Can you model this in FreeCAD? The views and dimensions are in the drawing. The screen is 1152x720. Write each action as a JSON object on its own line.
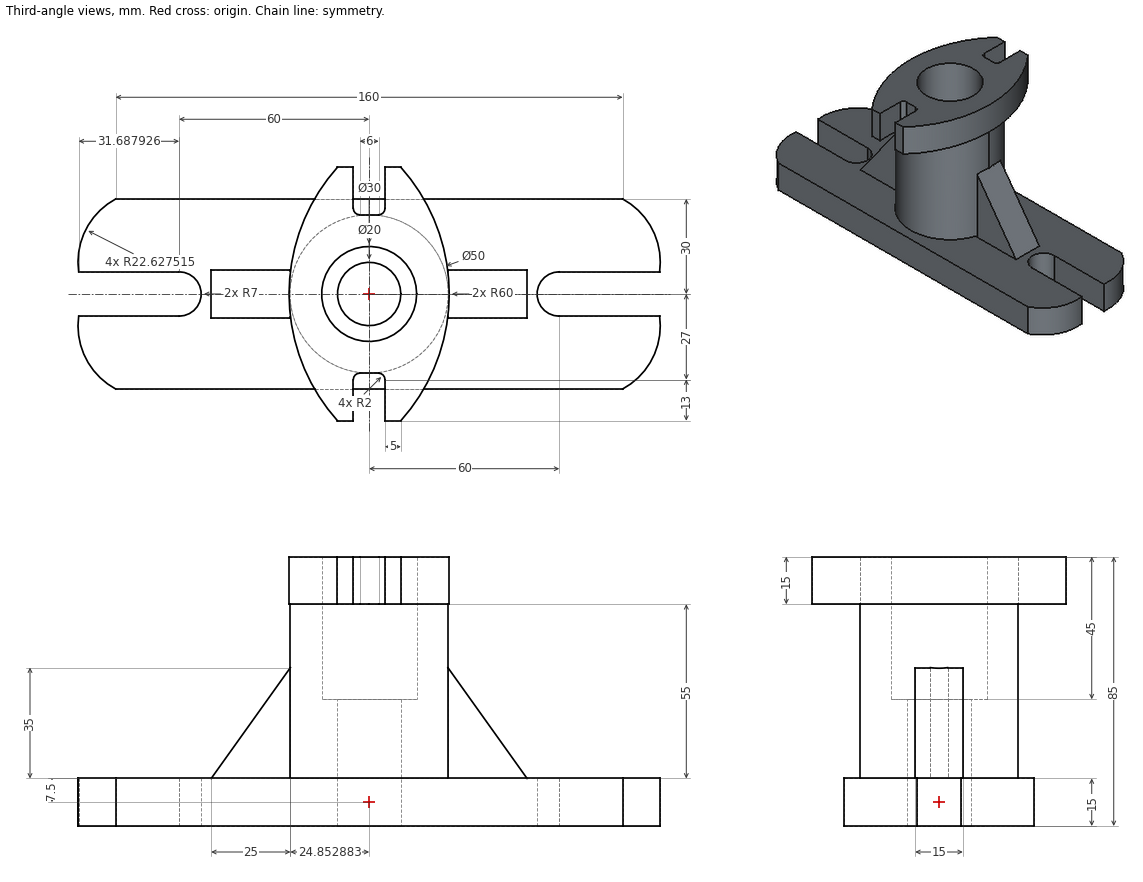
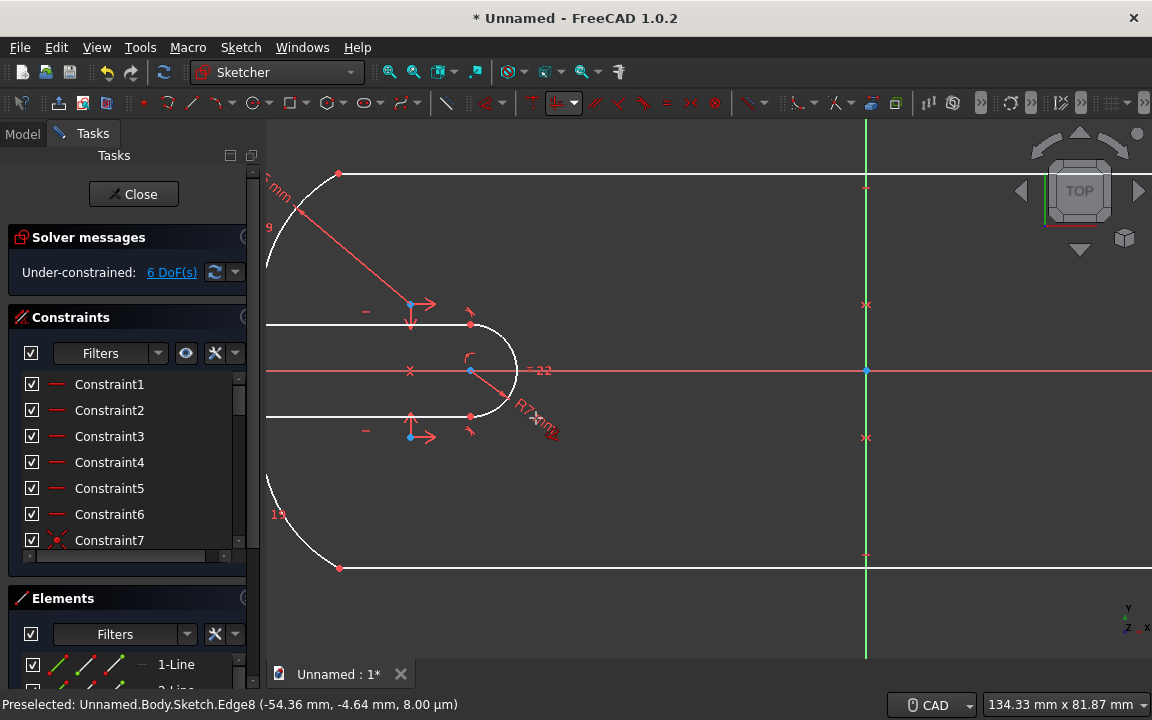
{"action": "left_click", "coordinate": [655, 174]}
{"action": "left_click", "coordinate": [663, 208]}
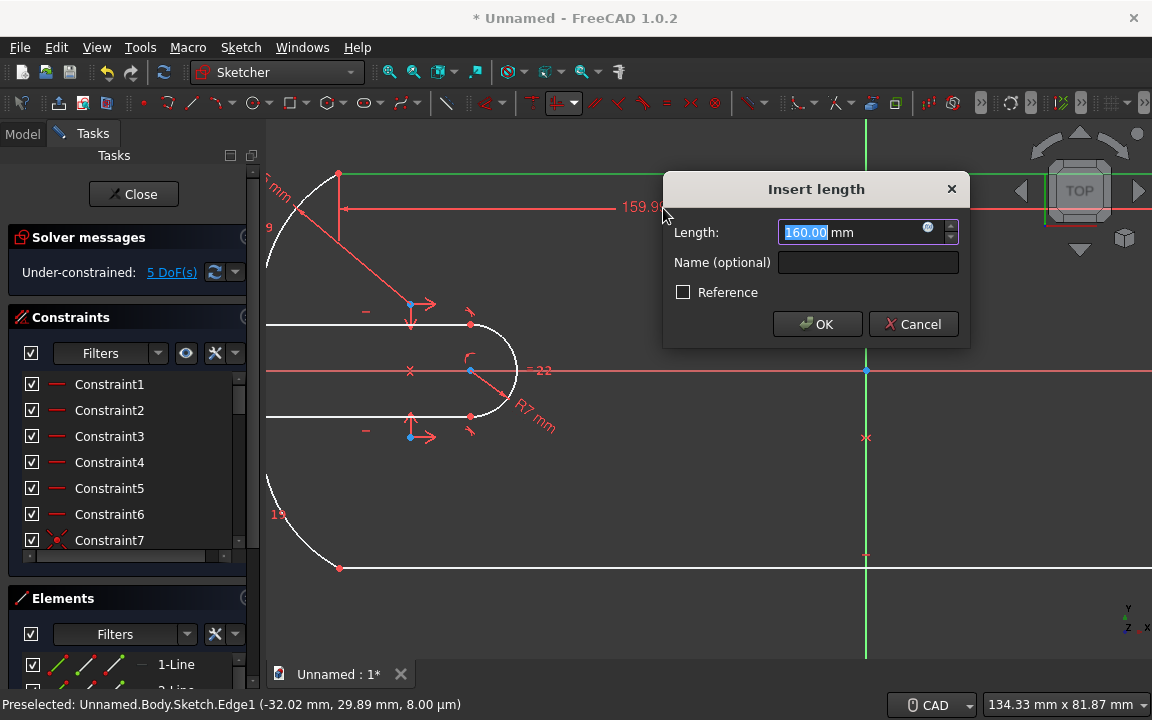
{"action": "type", "text": "160"}
{"action": "key", "text": "Return"}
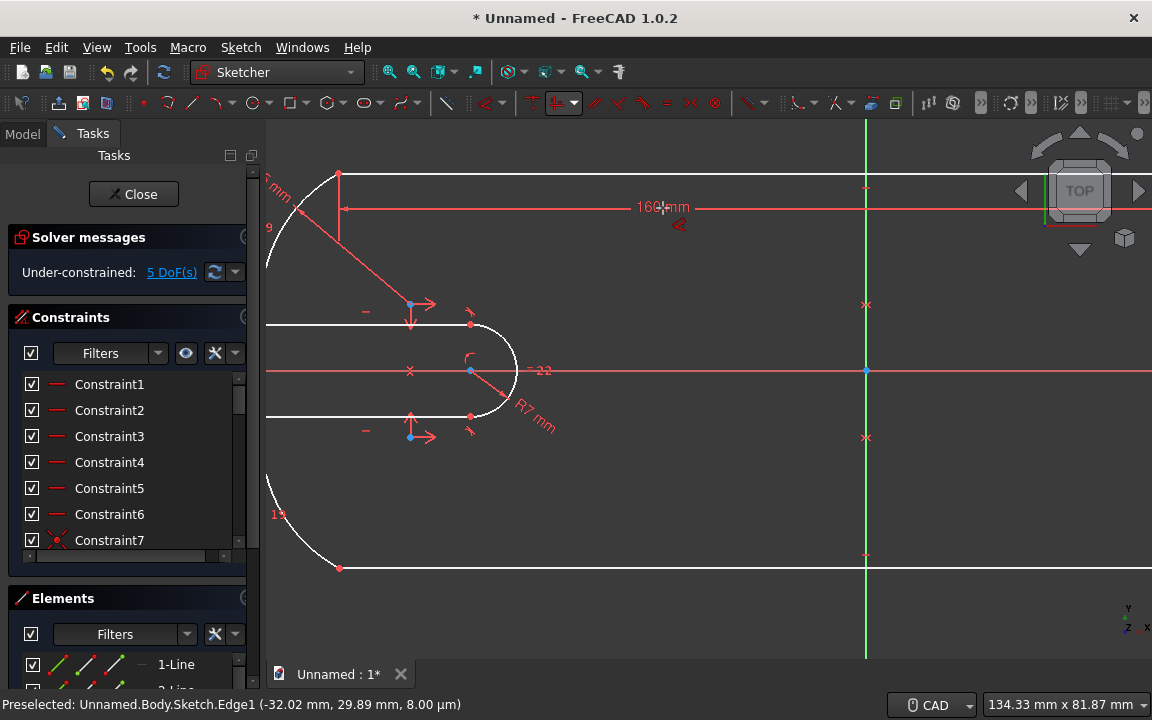
{"action": "left_click", "coordinate": [656, 568]}
{"action": "left_click", "coordinate": [663, 602]}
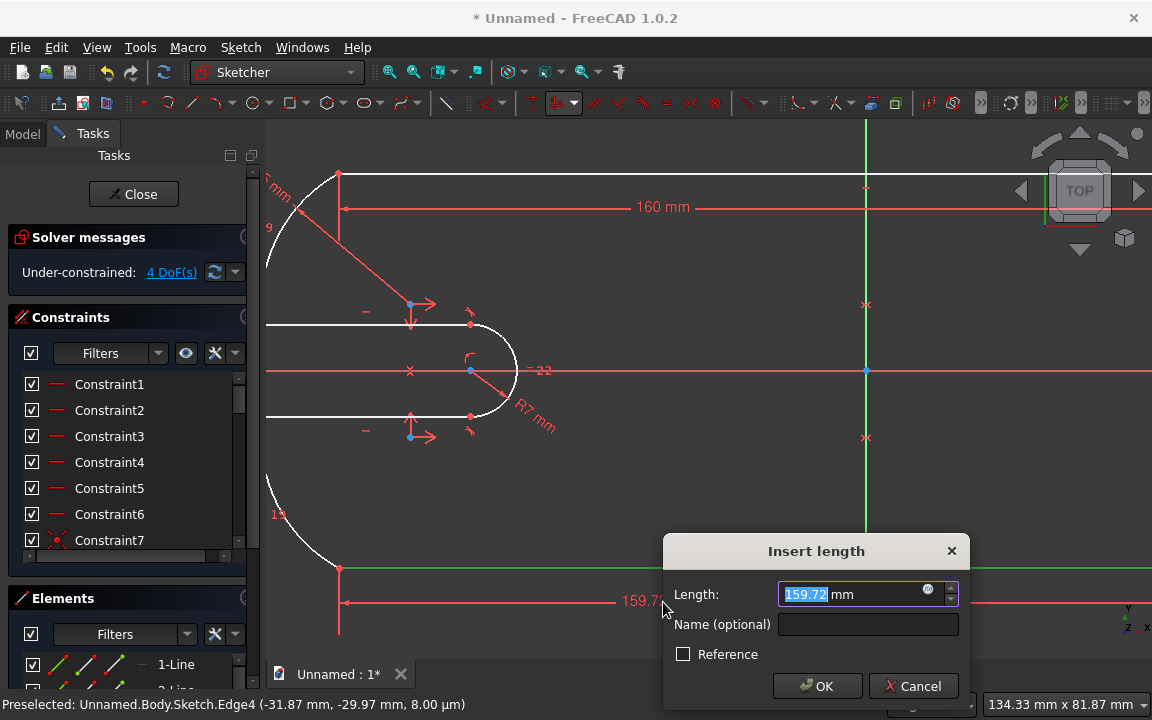
{"action": "type", "text": "160"}
{"action": "key", "text": "Return"}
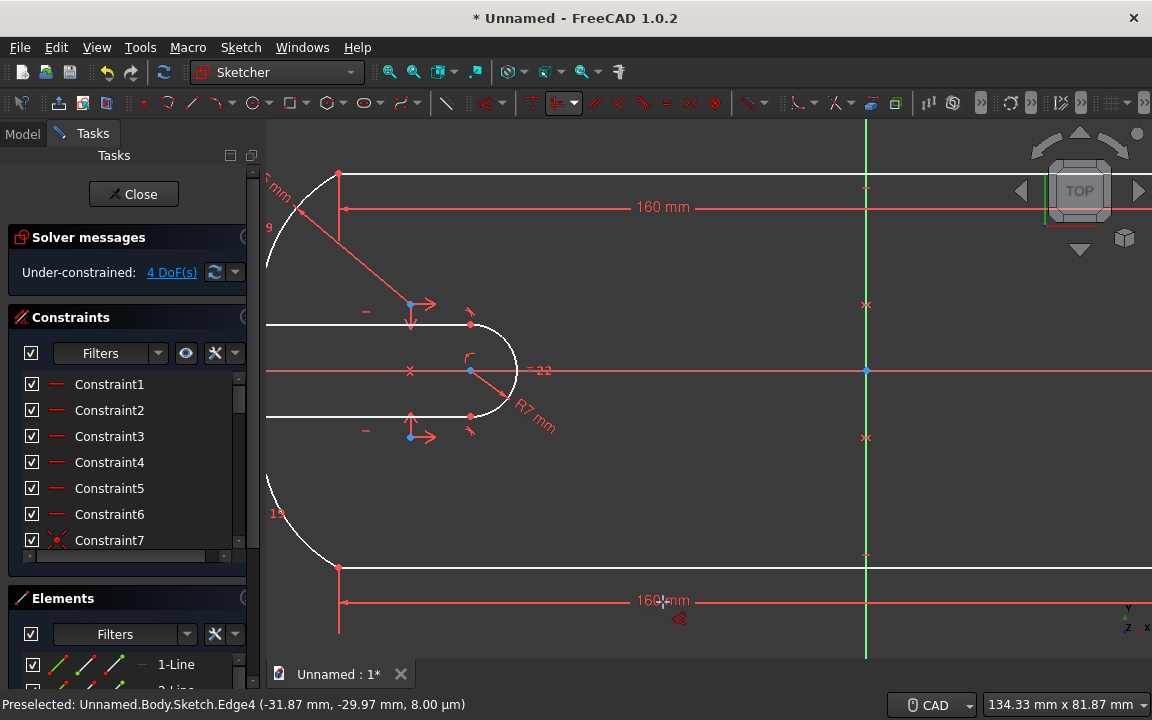
{"action": "scroll", "coordinate": [509, 400], "scroll_direction": "down", "scroll_amount": 5}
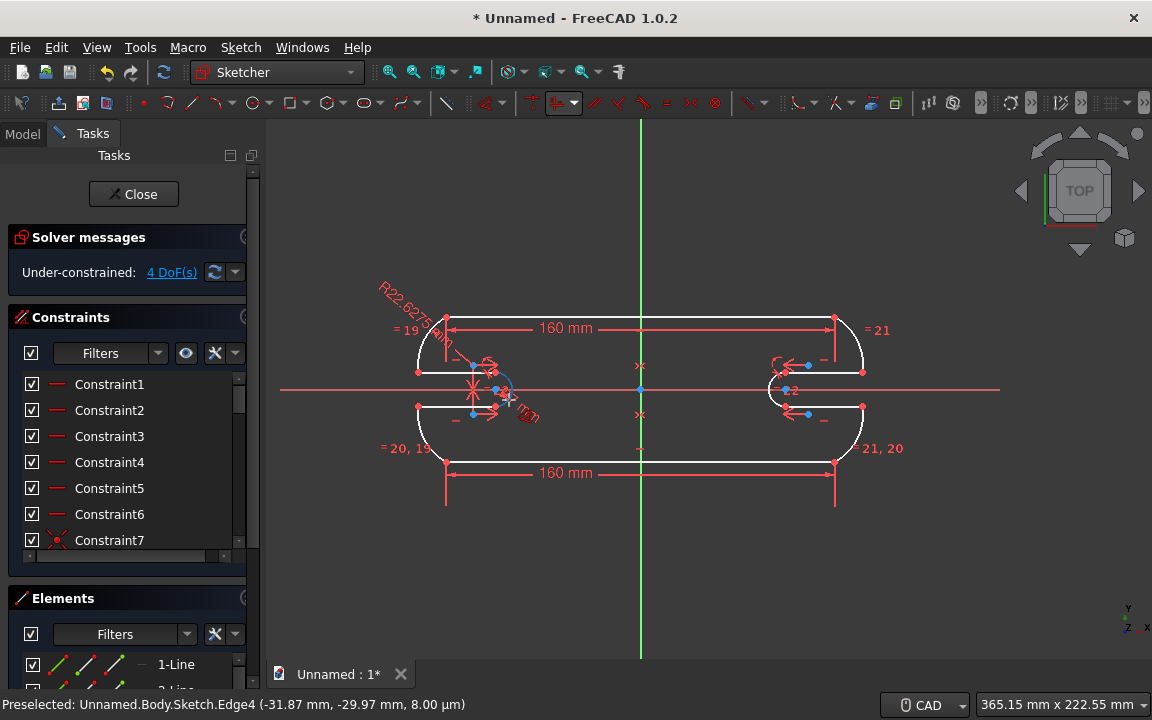
{"action": "left_click", "coordinate": [835, 317]}
{"action": "left_click", "coordinate": [869, 328]}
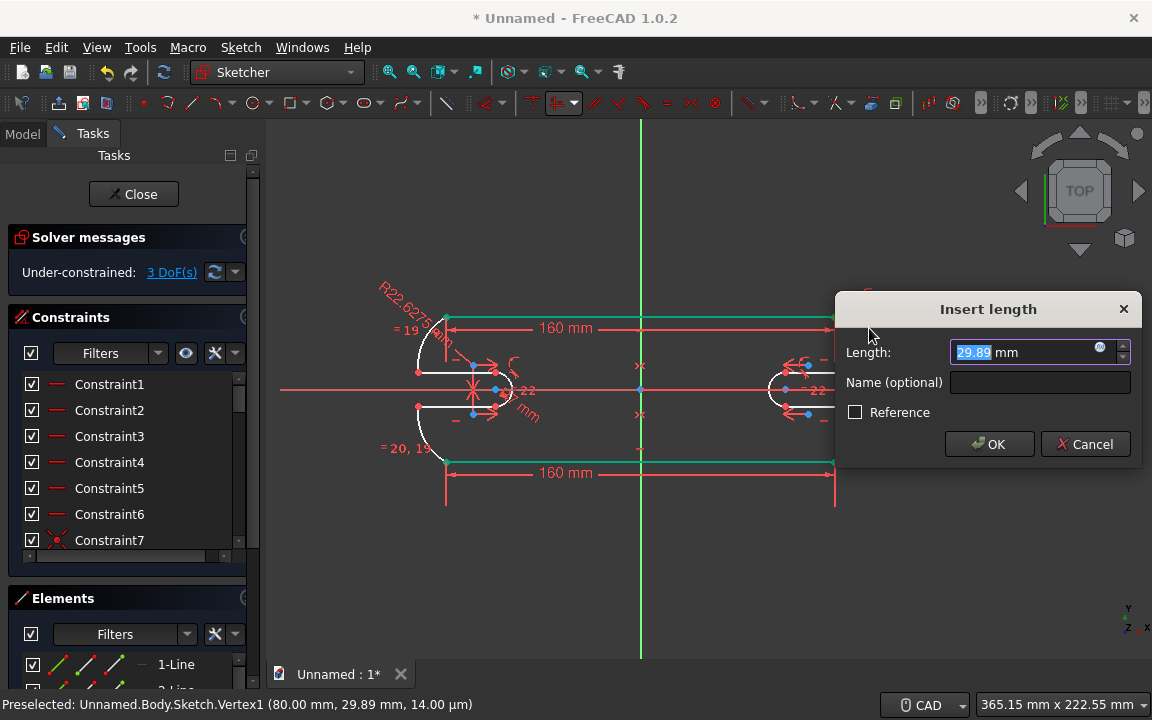
{"action": "type", "text": "30"}
{"action": "key", "text": "Return"}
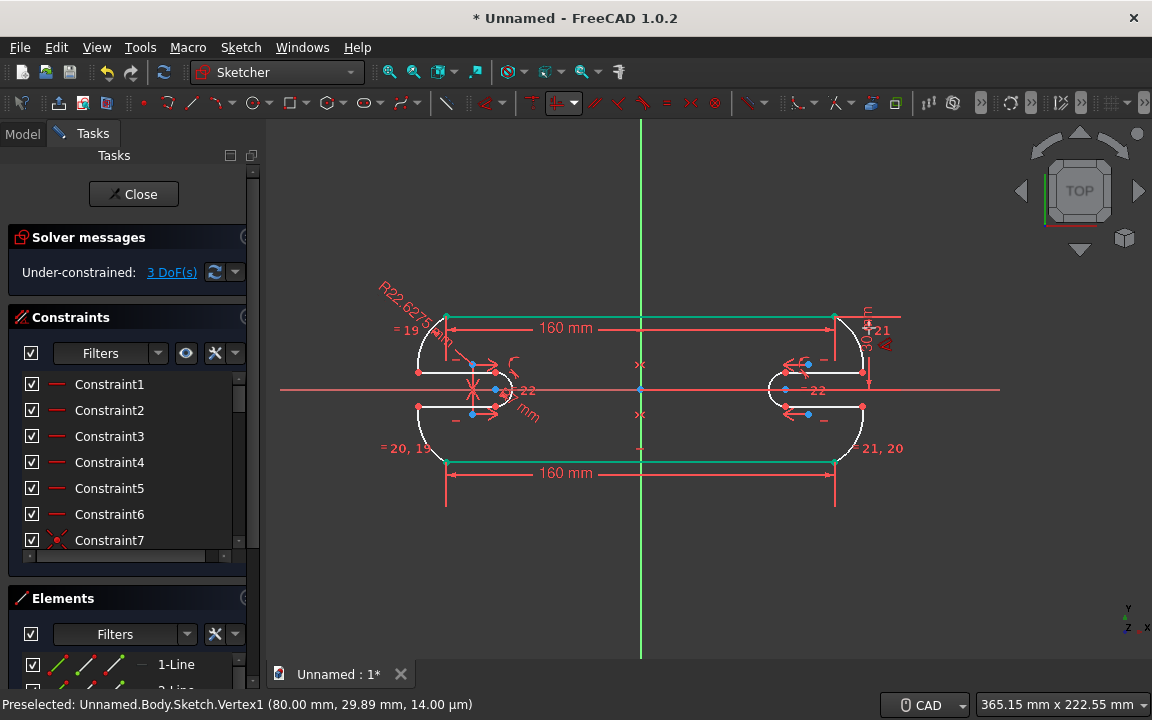
{"action": "left_click", "coordinate": [495, 373]}
{"action": "left_click", "coordinate": [601, 424]}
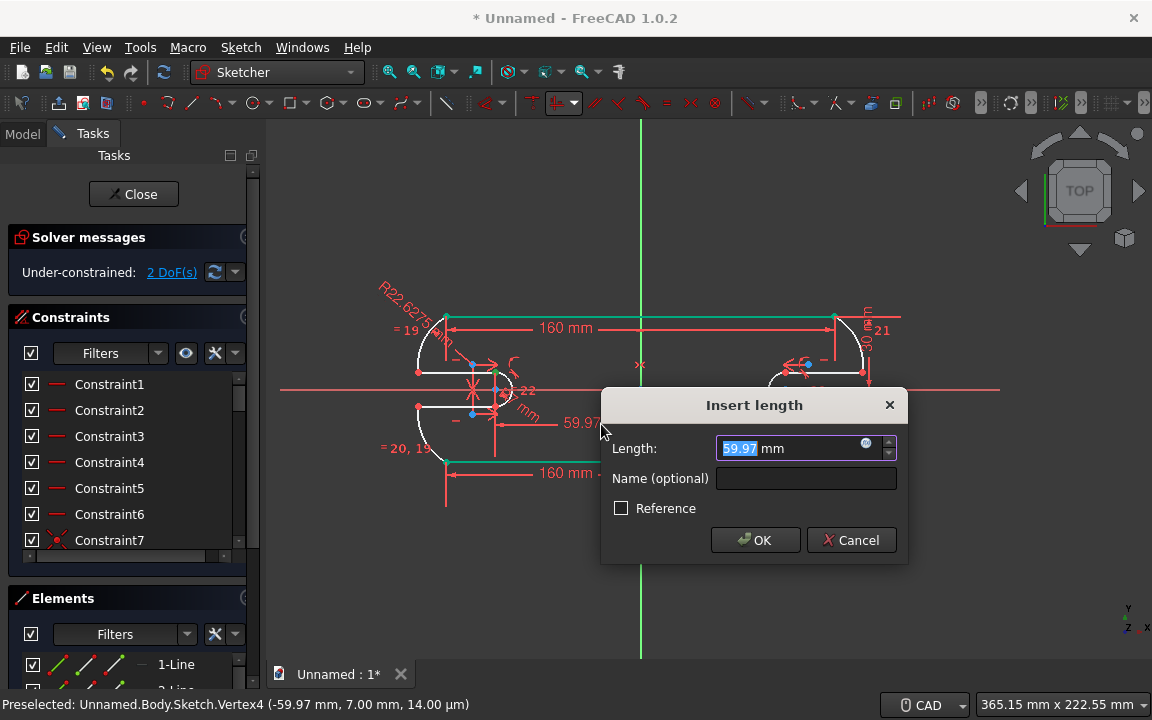
{"action": "type", "text": "60"}
{"action": "key", "text": "Return"}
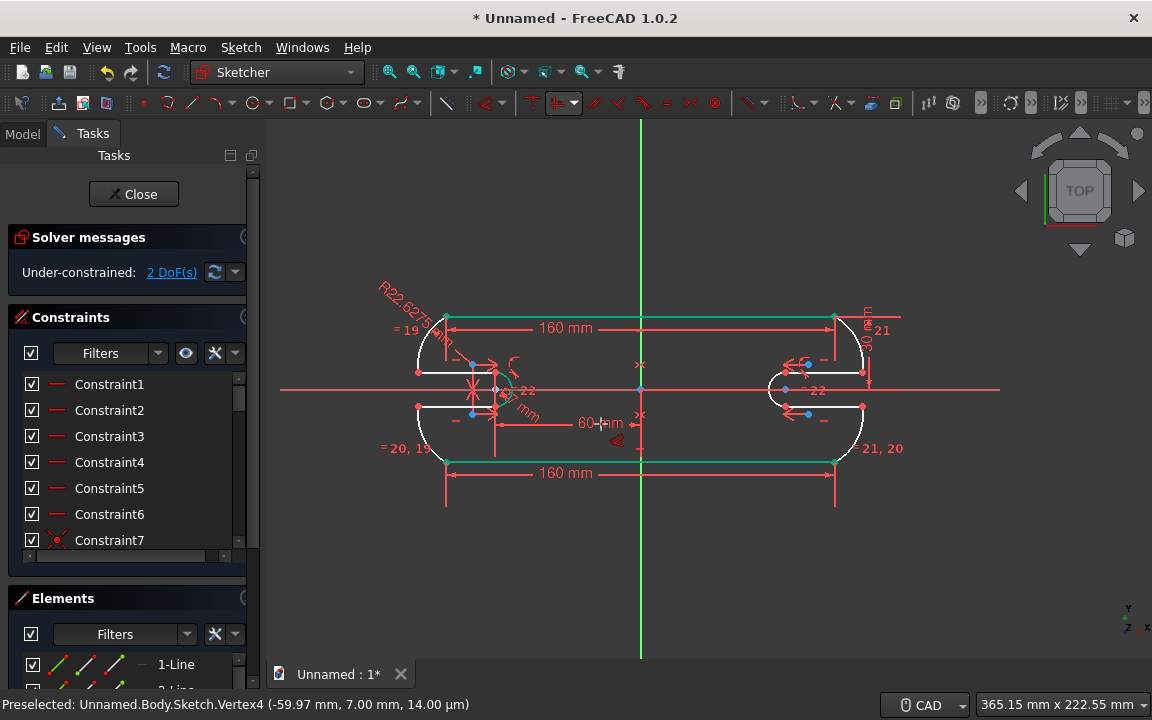
{"action": "left_click", "coordinate": [786, 407]}
{"action": "left_click", "coordinate": [713, 441]}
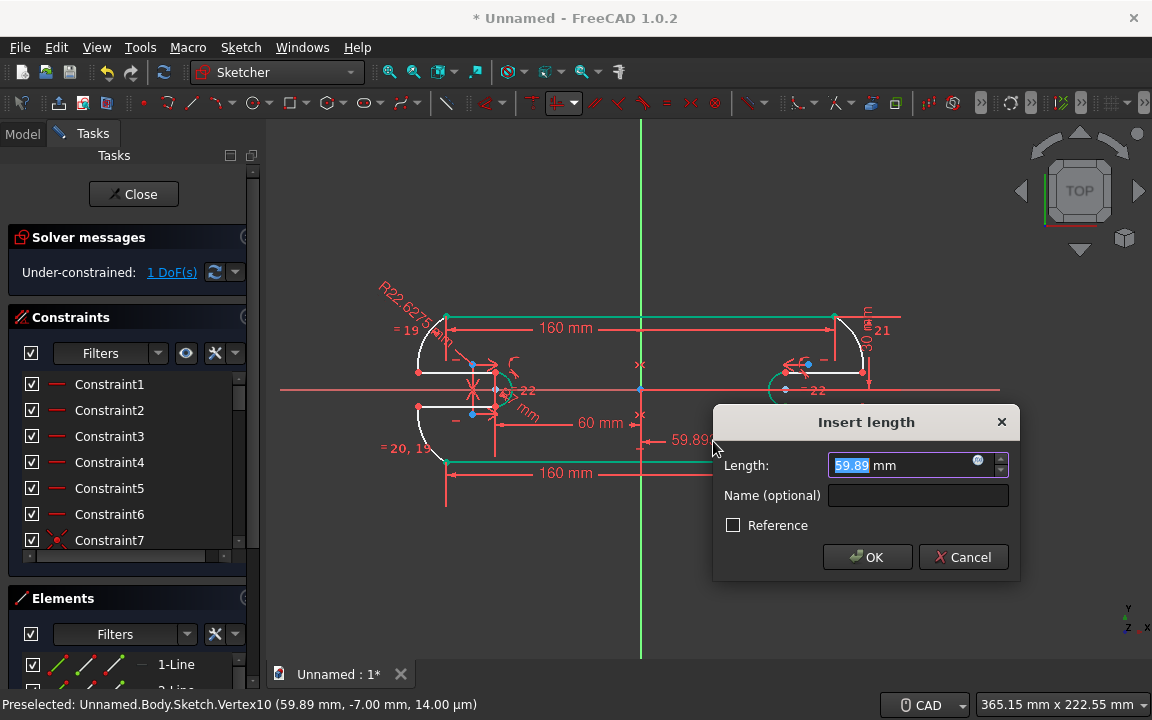
{"action": "type", "text": "60"}
{"action": "key", "text": "Return"}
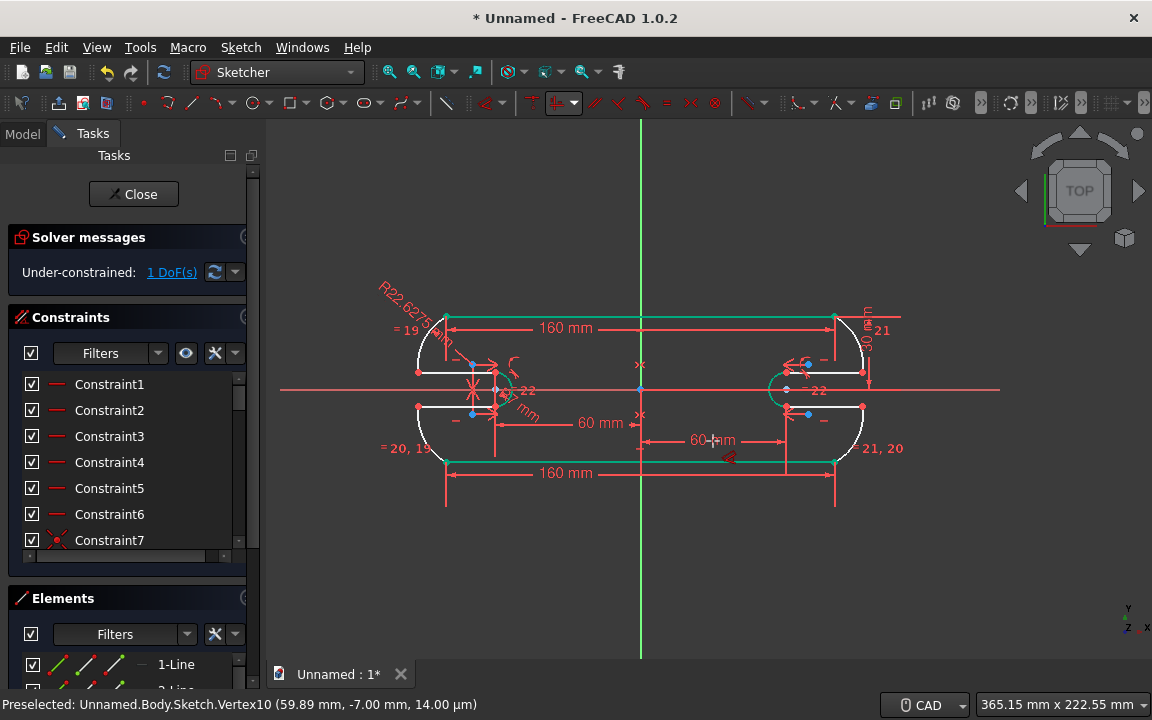
{"action": "left_click", "coordinate": [442, 373]}
{"action": "left_click", "coordinate": [457, 339]}